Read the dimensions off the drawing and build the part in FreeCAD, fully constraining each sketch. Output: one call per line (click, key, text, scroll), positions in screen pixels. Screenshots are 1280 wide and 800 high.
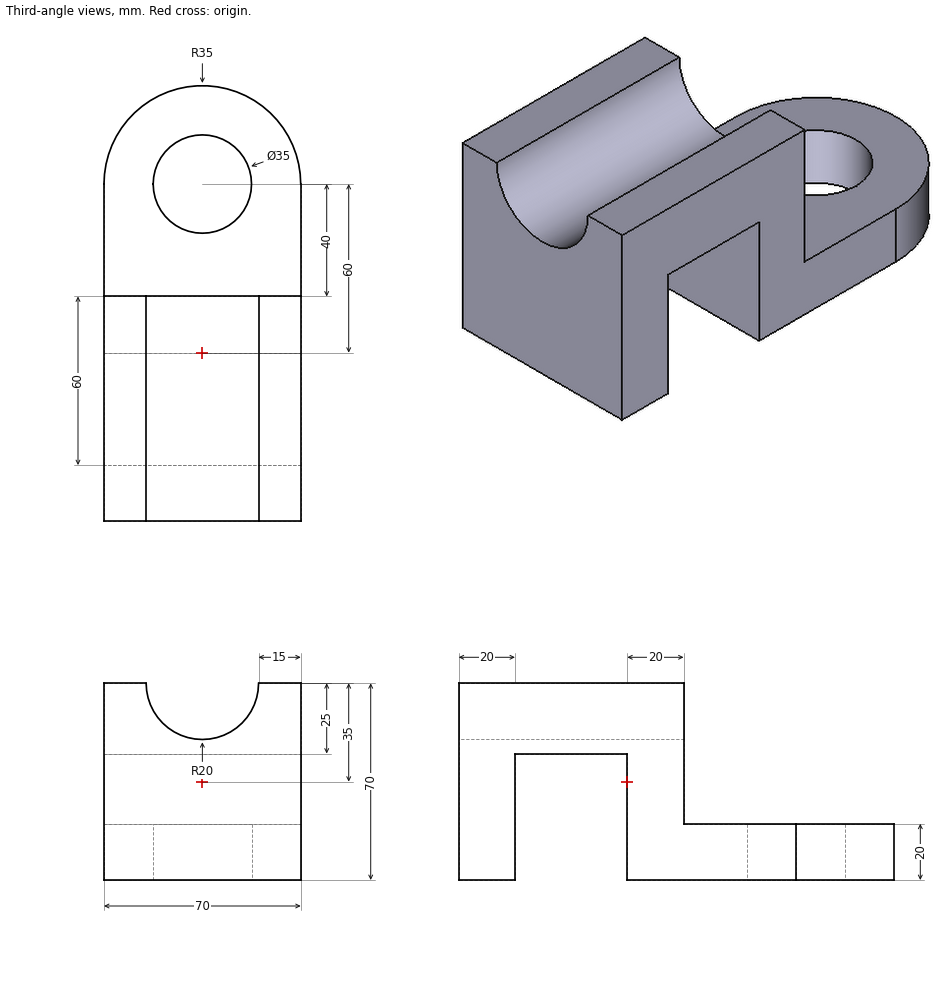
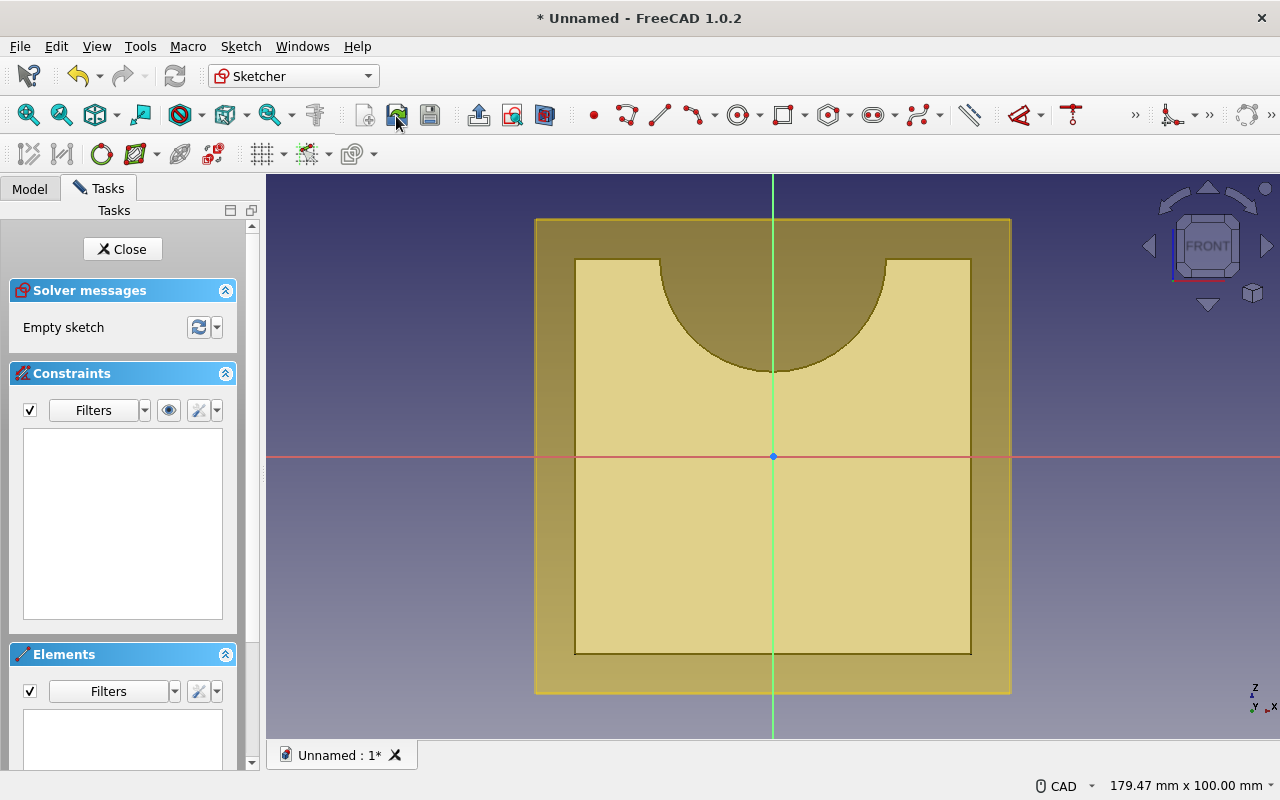
scroll(912, 202, up, 2)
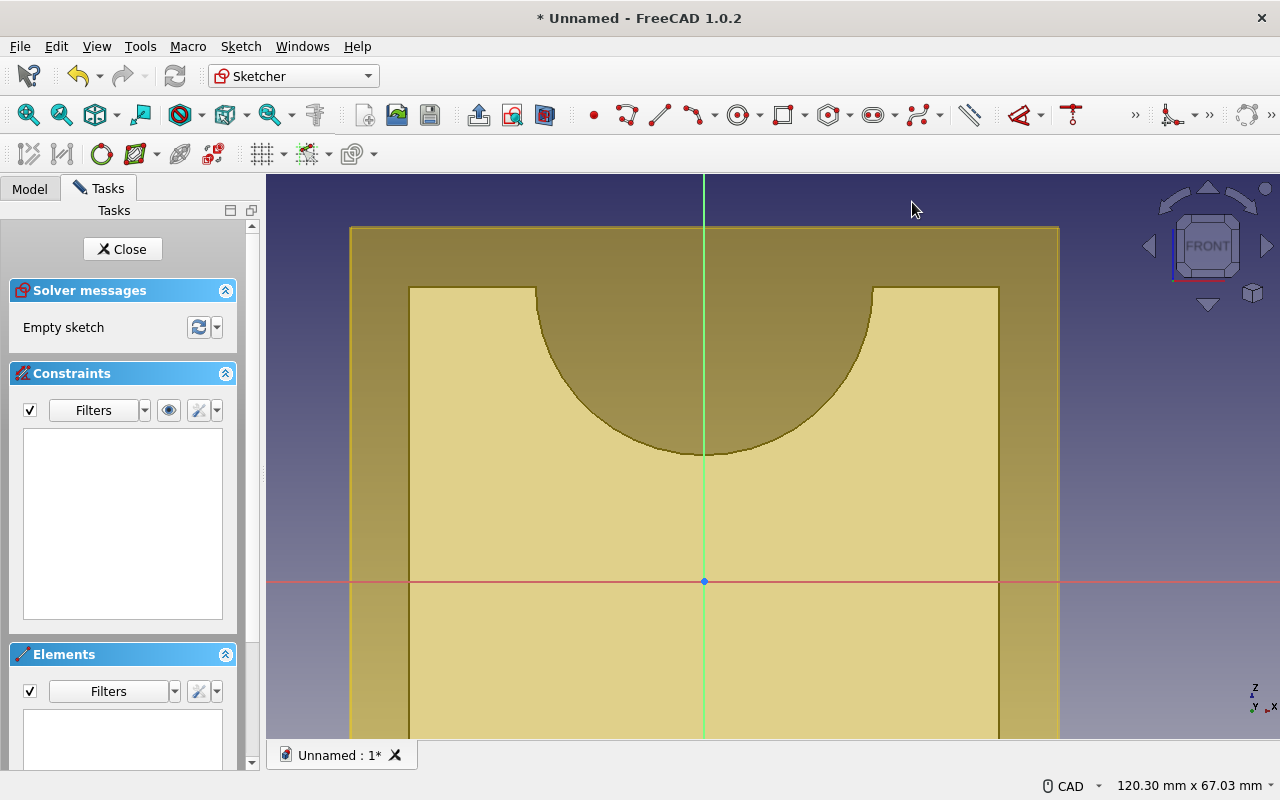
click(627, 116)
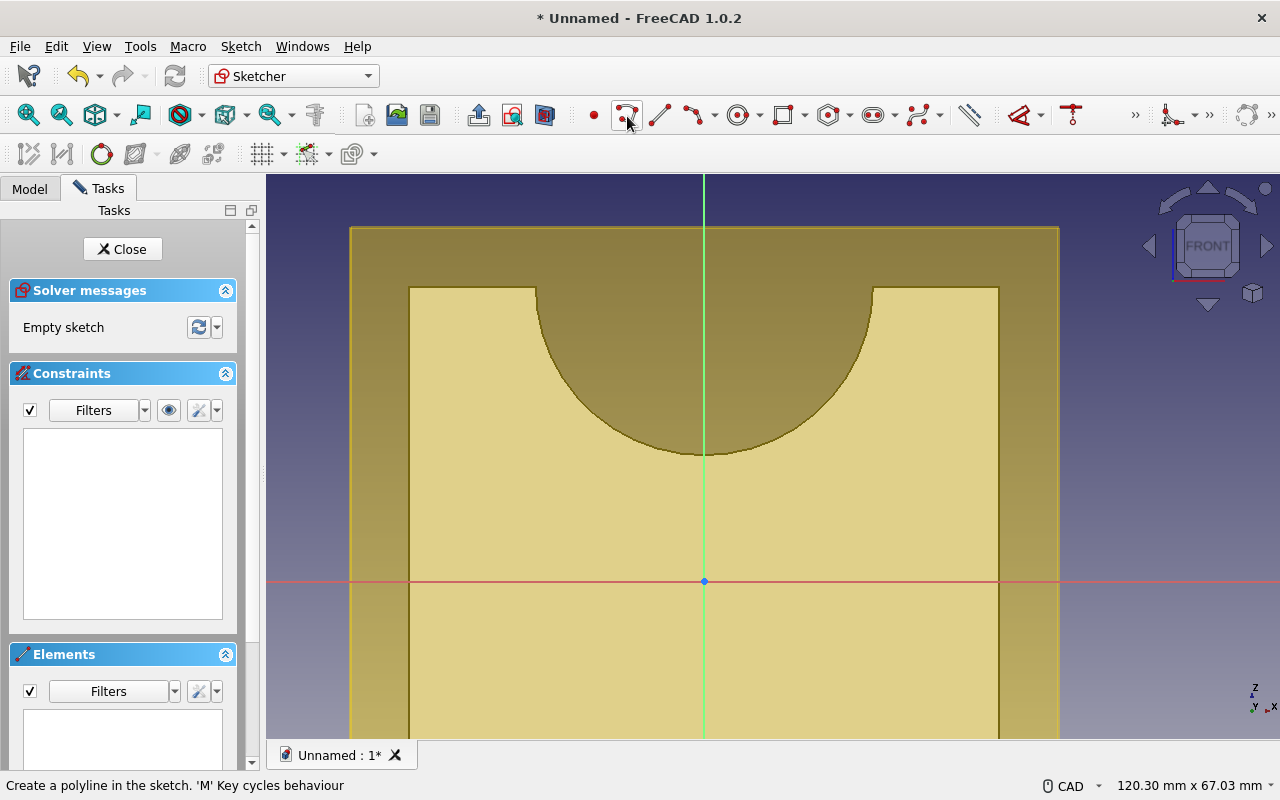
click(873, 287)
click(999, 287)
click(999, 497)
click(409, 497)
click(409, 287)
click(536, 287)
right_click(536, 287)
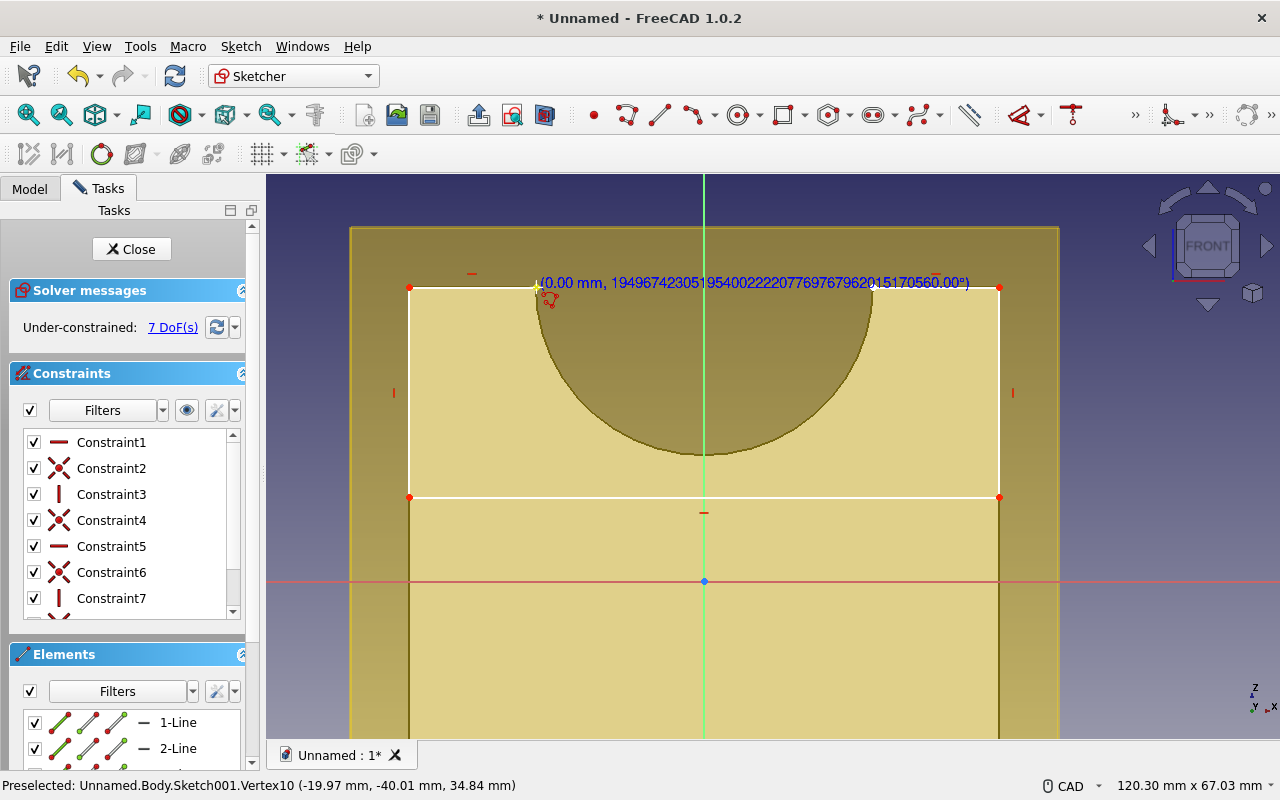
click(692, 116)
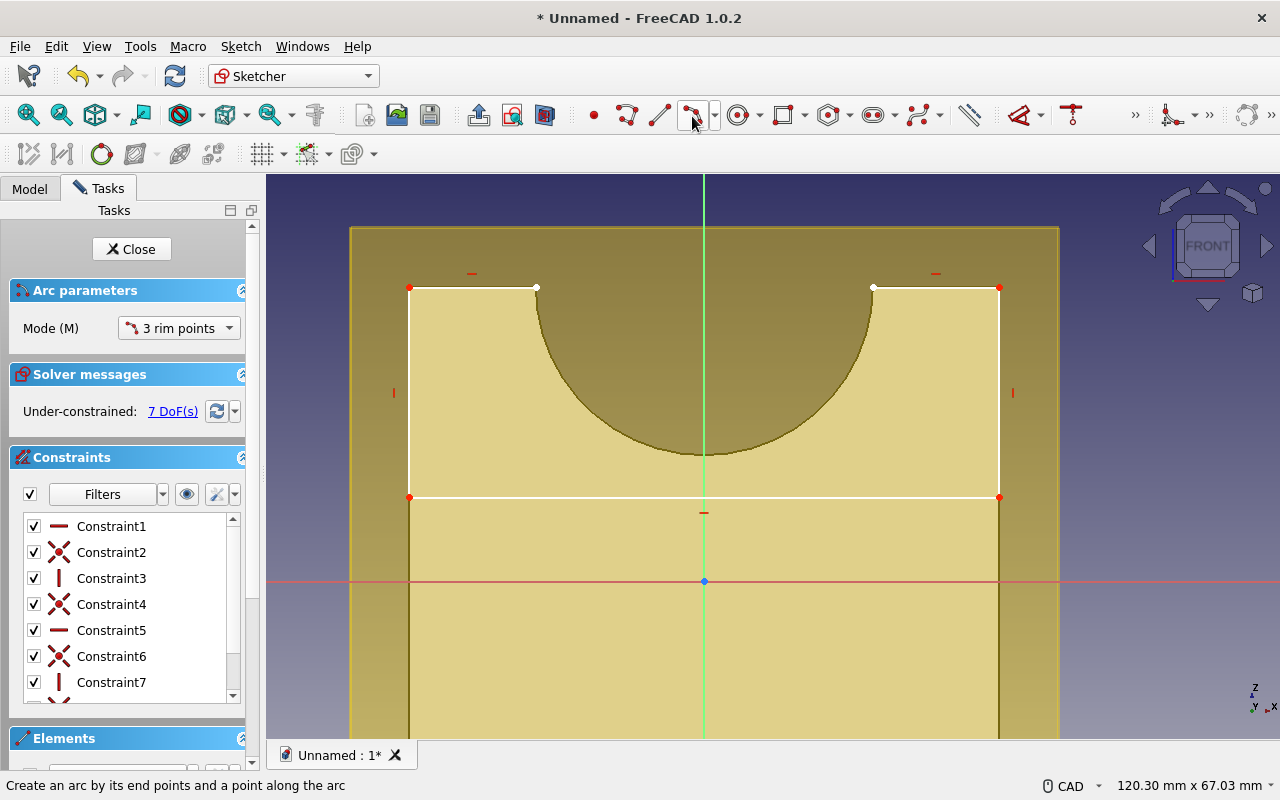
click(536, 288)
click(873, 288)
click(652, 447)
key(Escape)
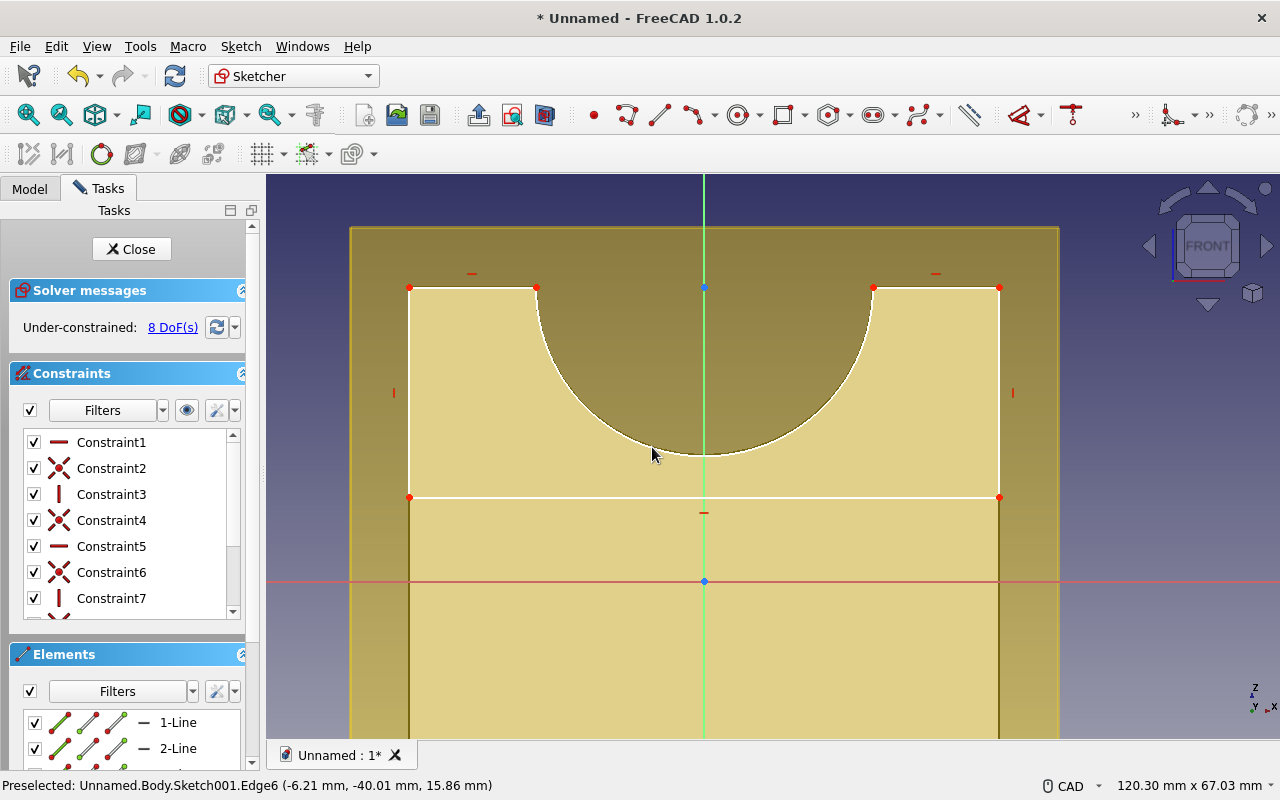
click(705, 288)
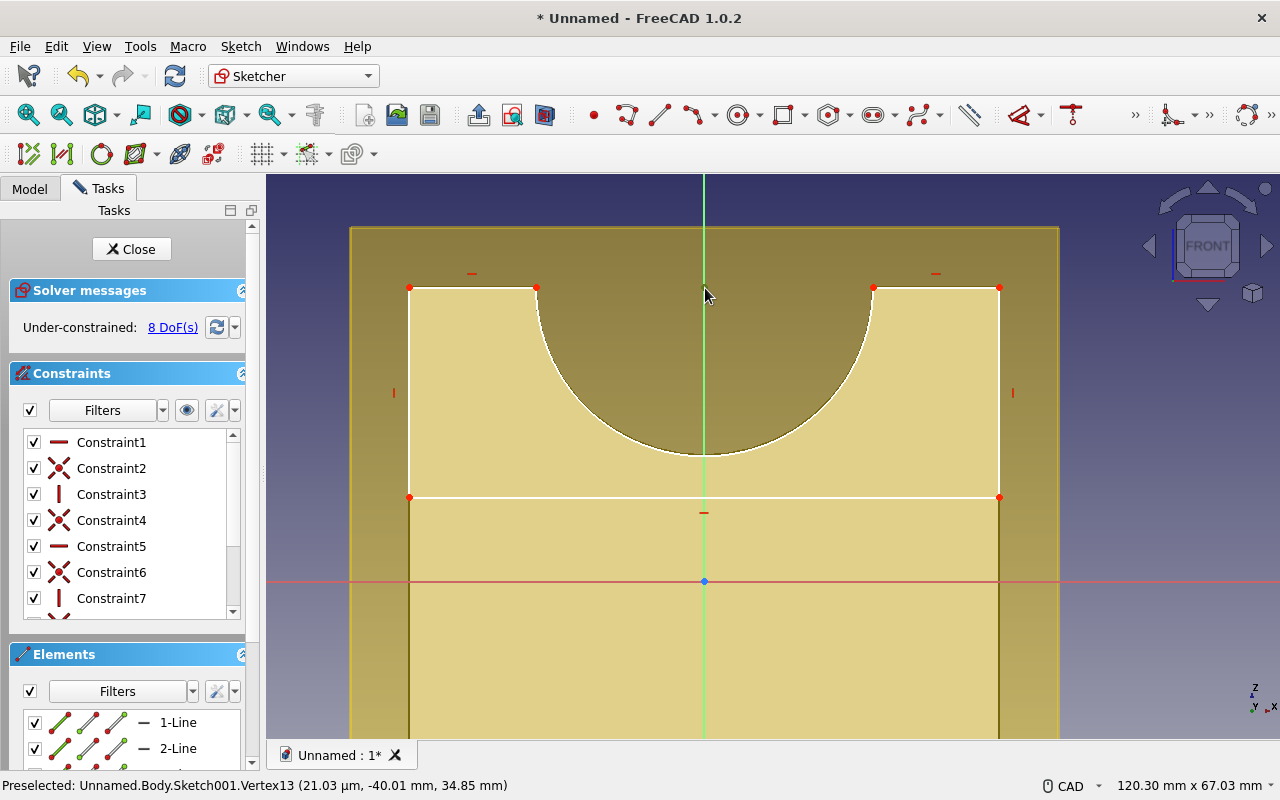
click(704, 675)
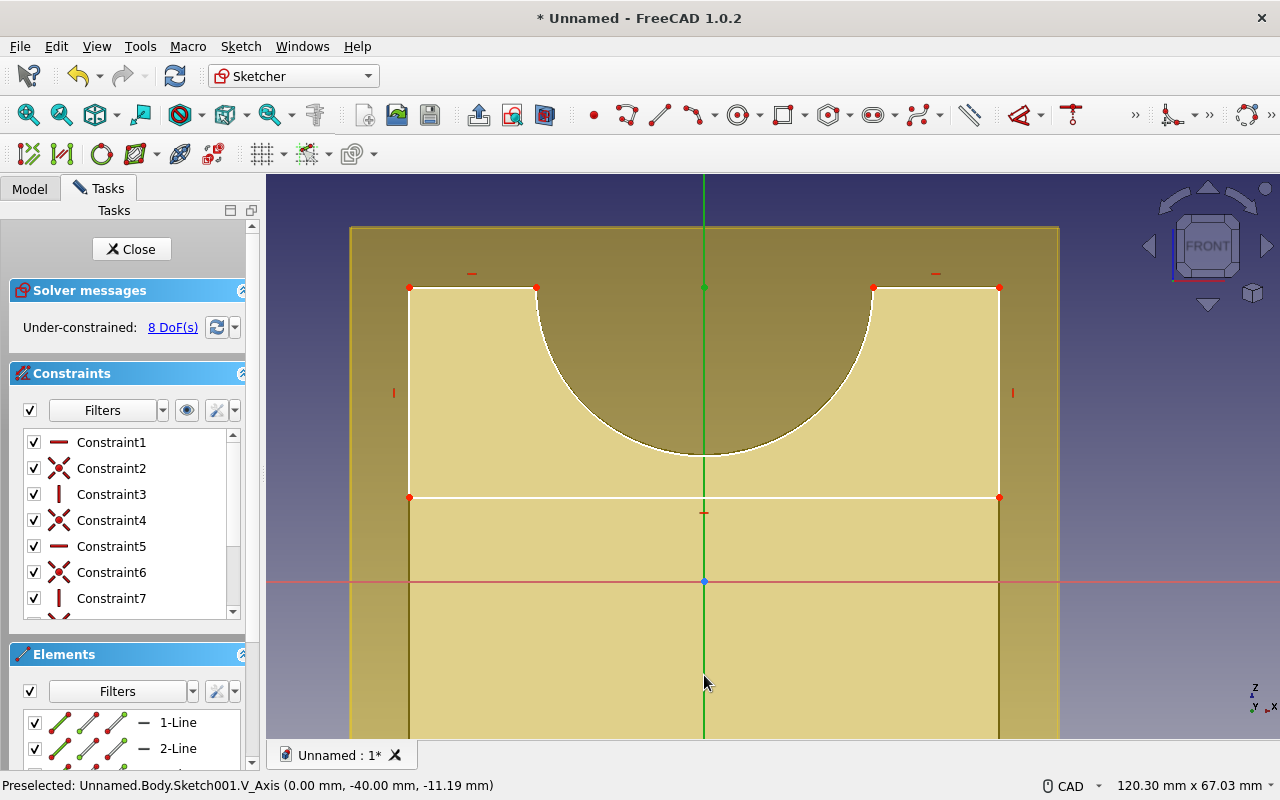
click(1071, 116)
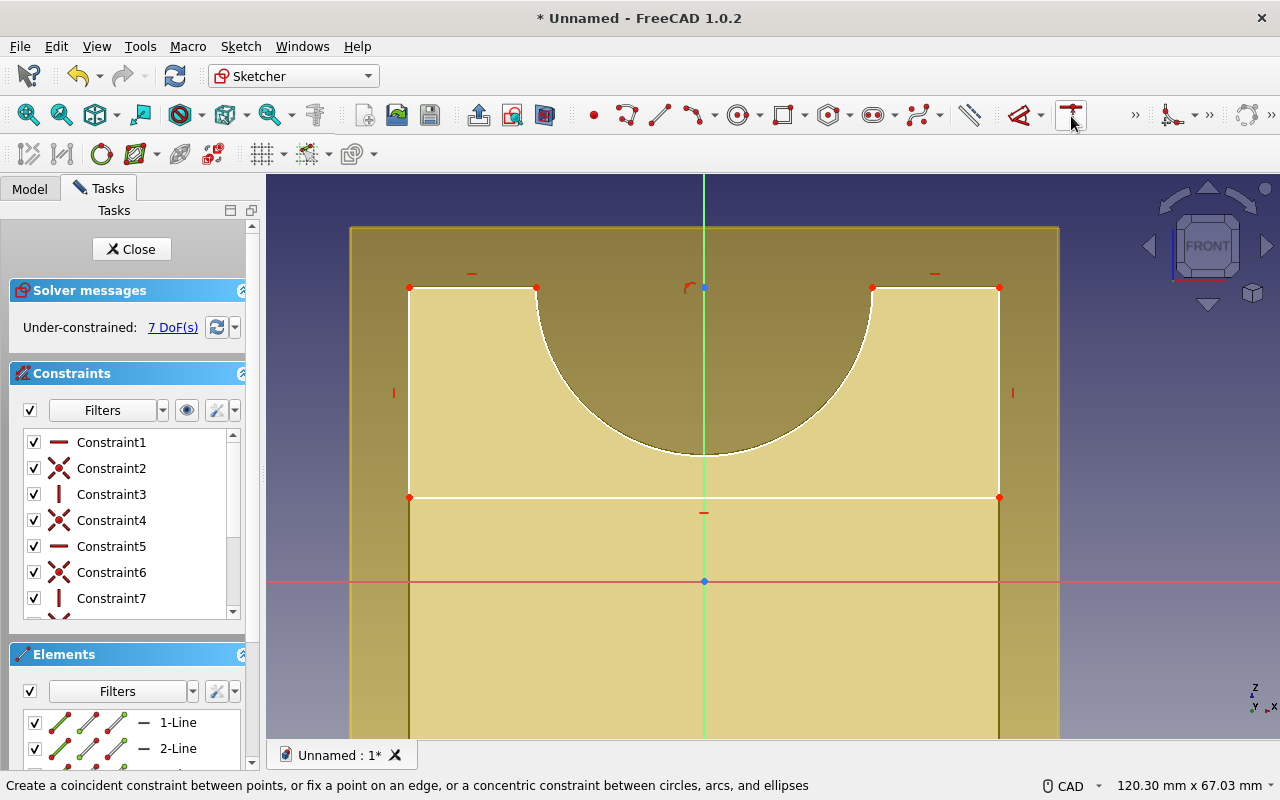
key(d)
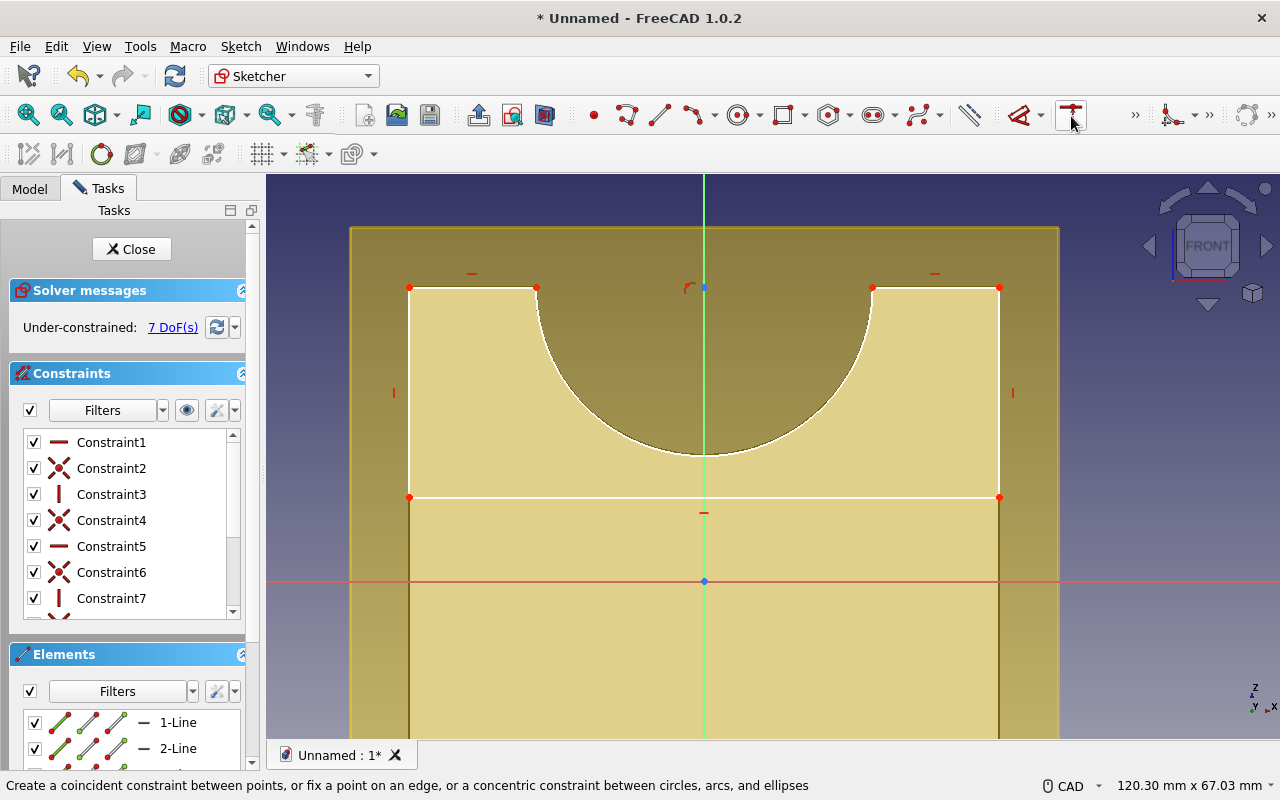
click(605, 424)
click(586, 450)